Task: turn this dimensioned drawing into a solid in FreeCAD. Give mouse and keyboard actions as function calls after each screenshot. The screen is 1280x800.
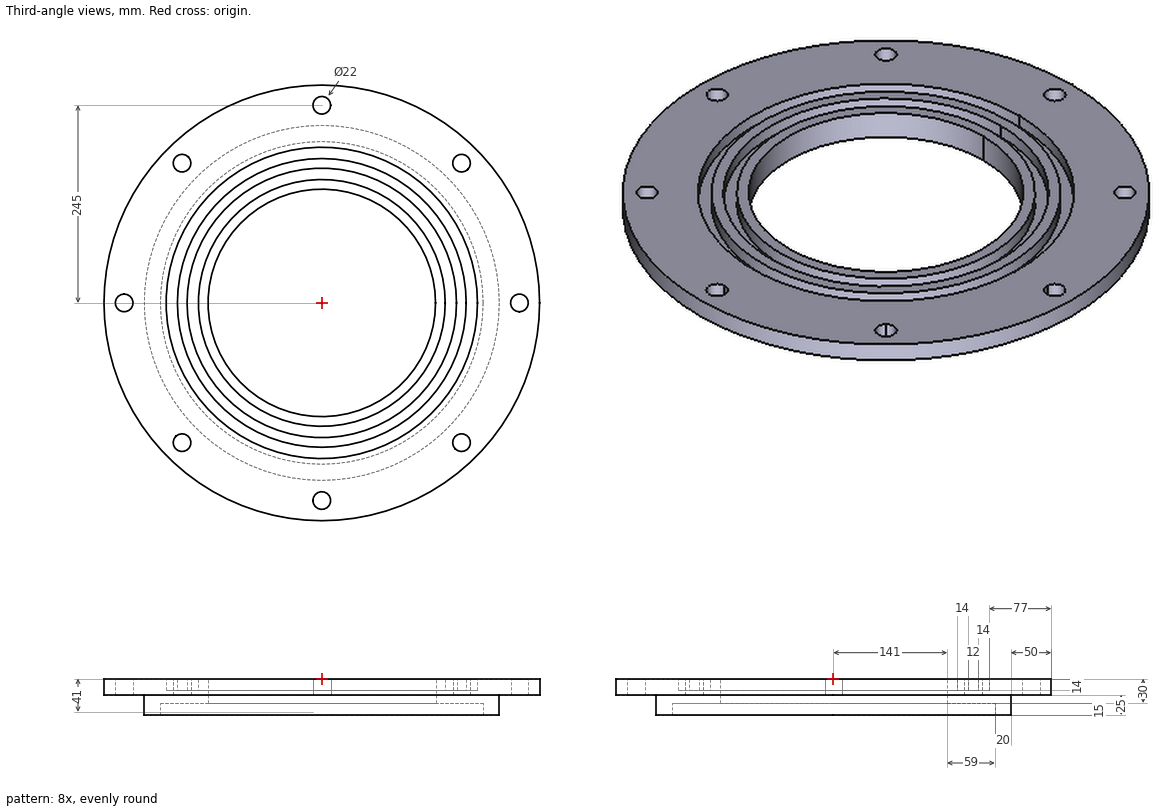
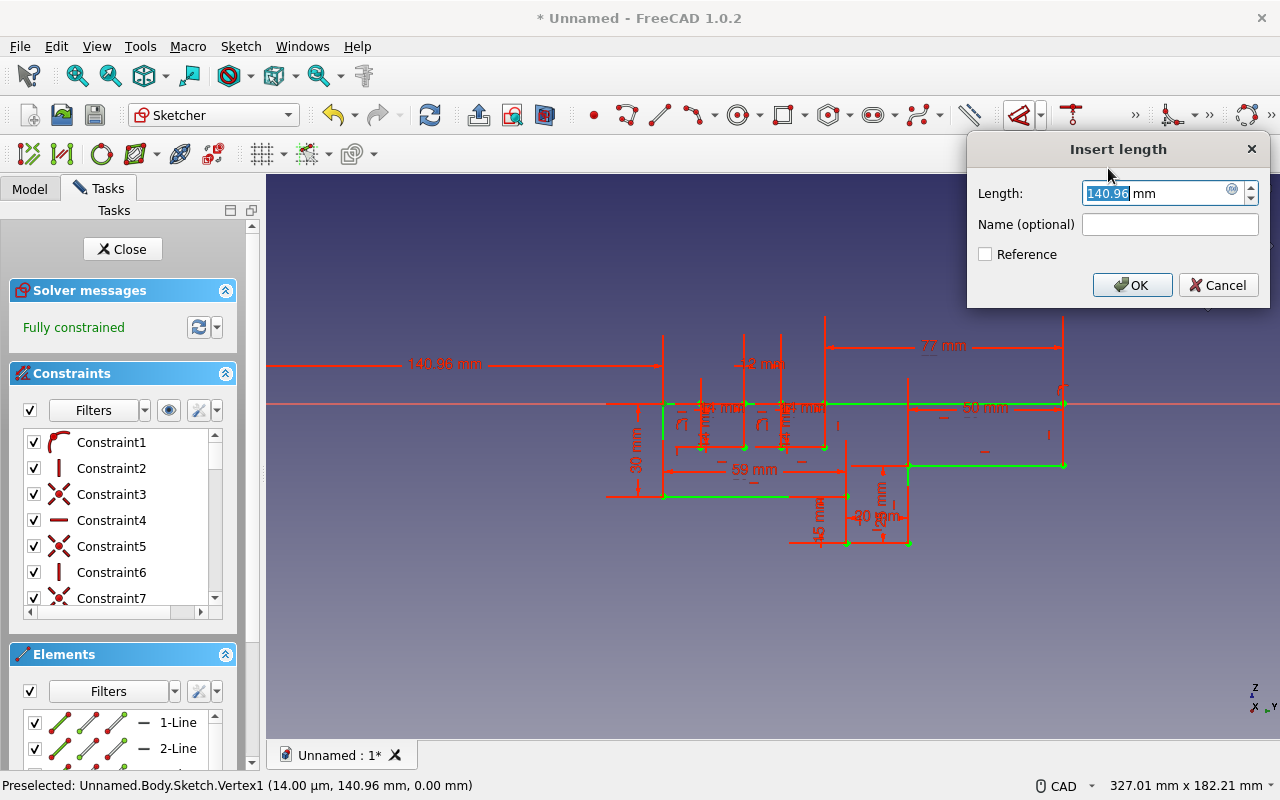
text(141)
key(Return)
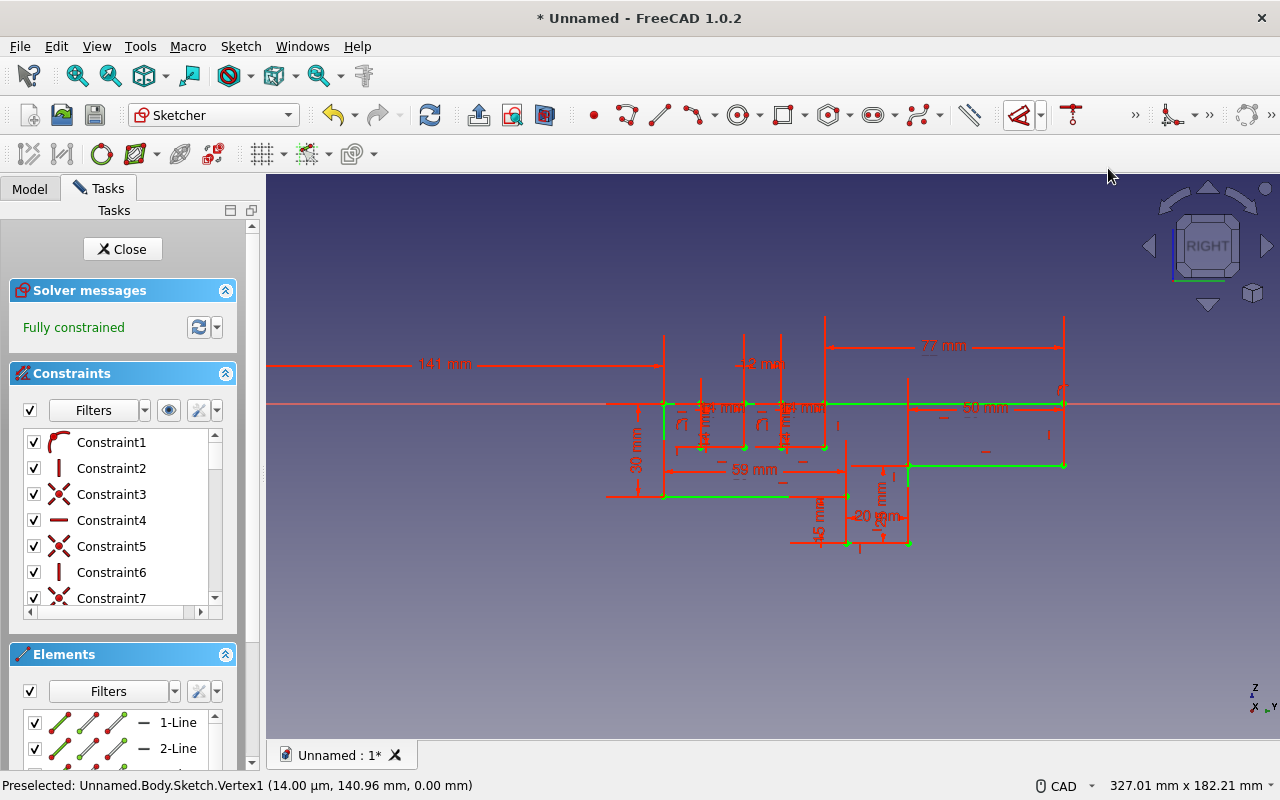
click(123, 249)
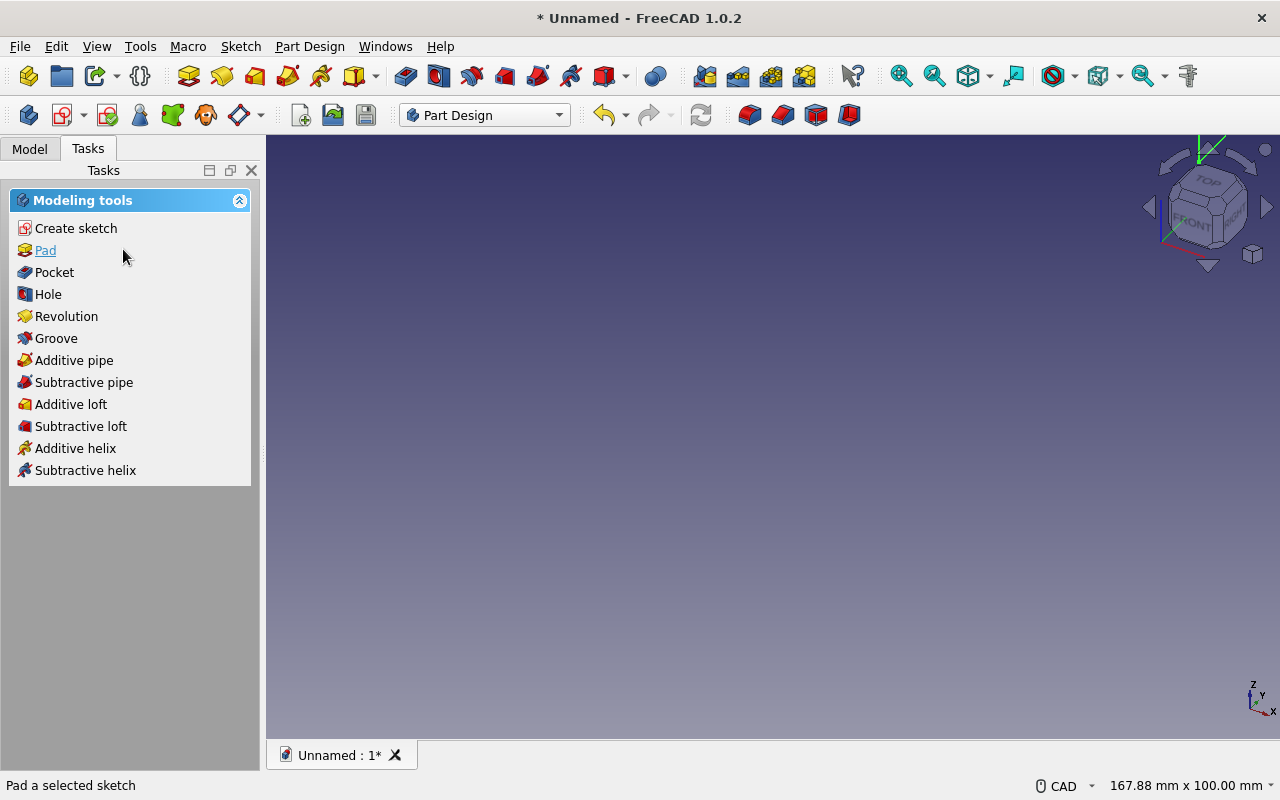
click(222, 76)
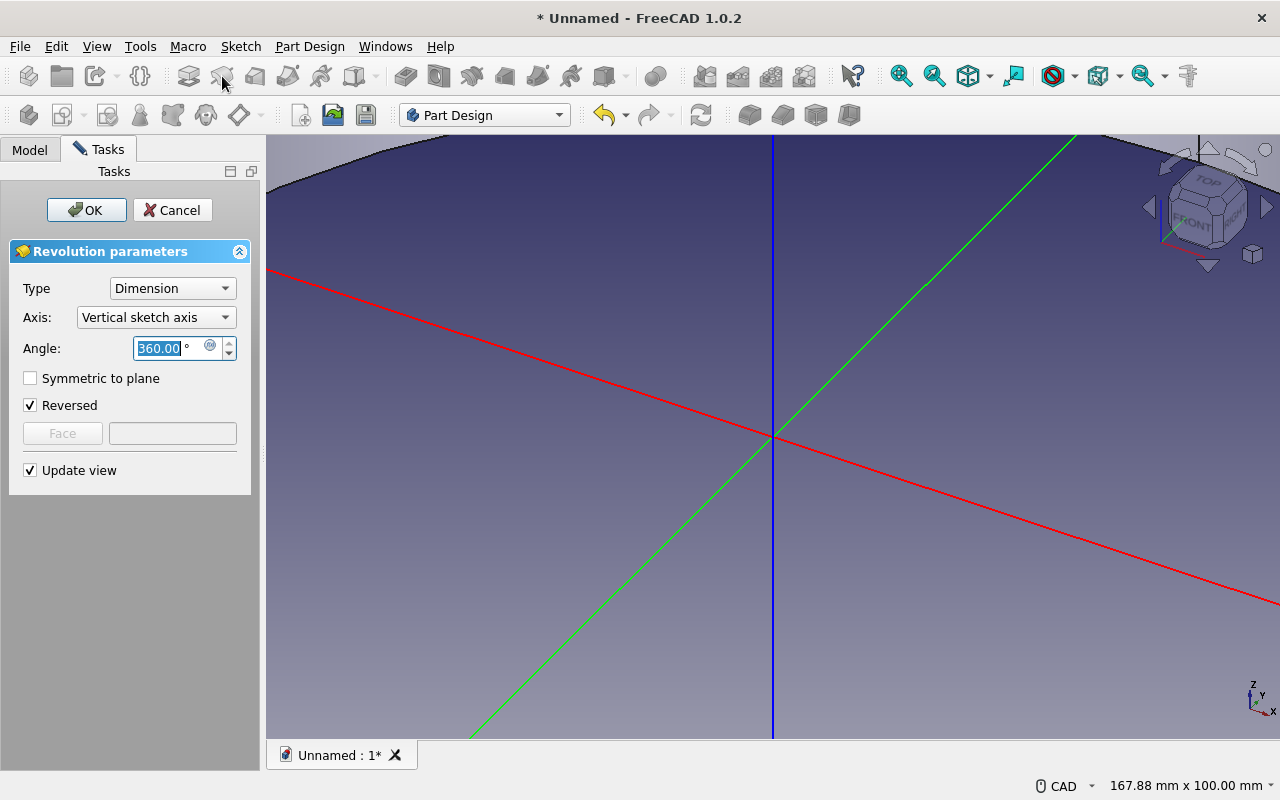
click(87, 210)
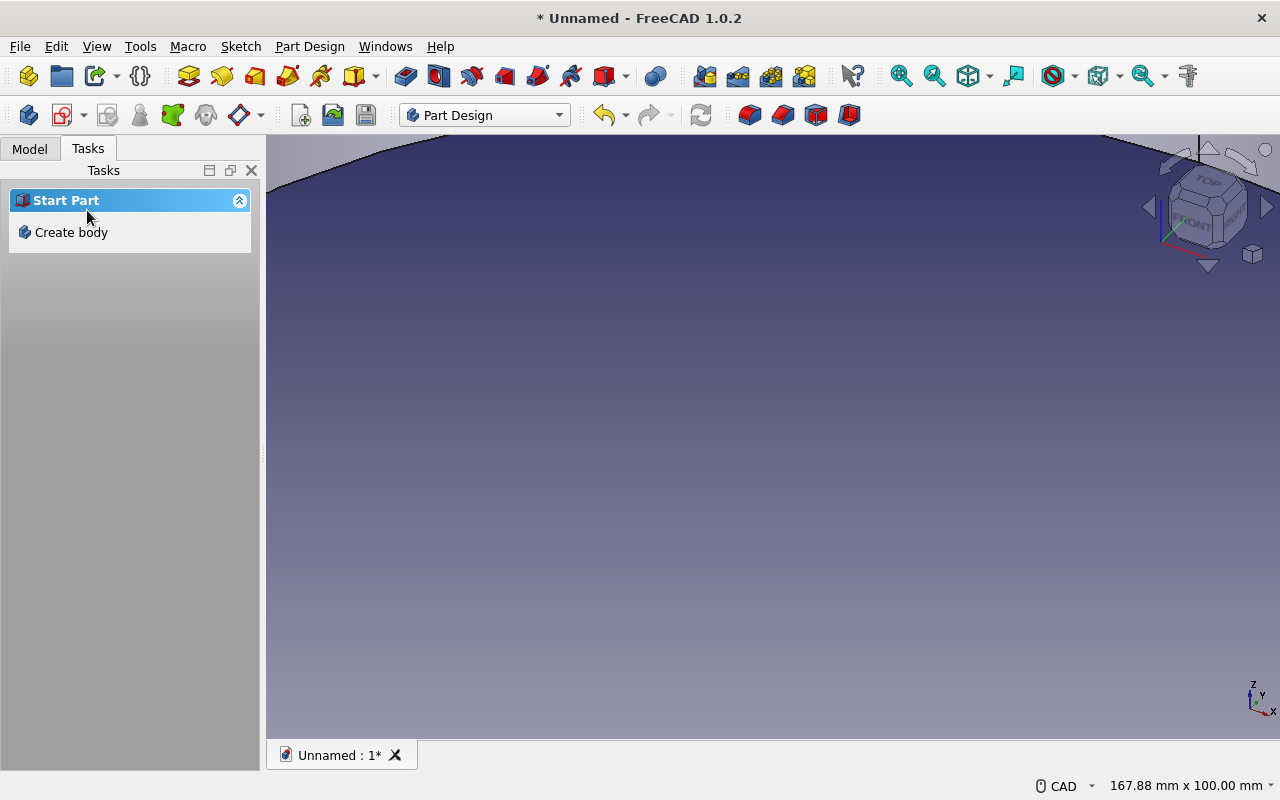
click(902, 76)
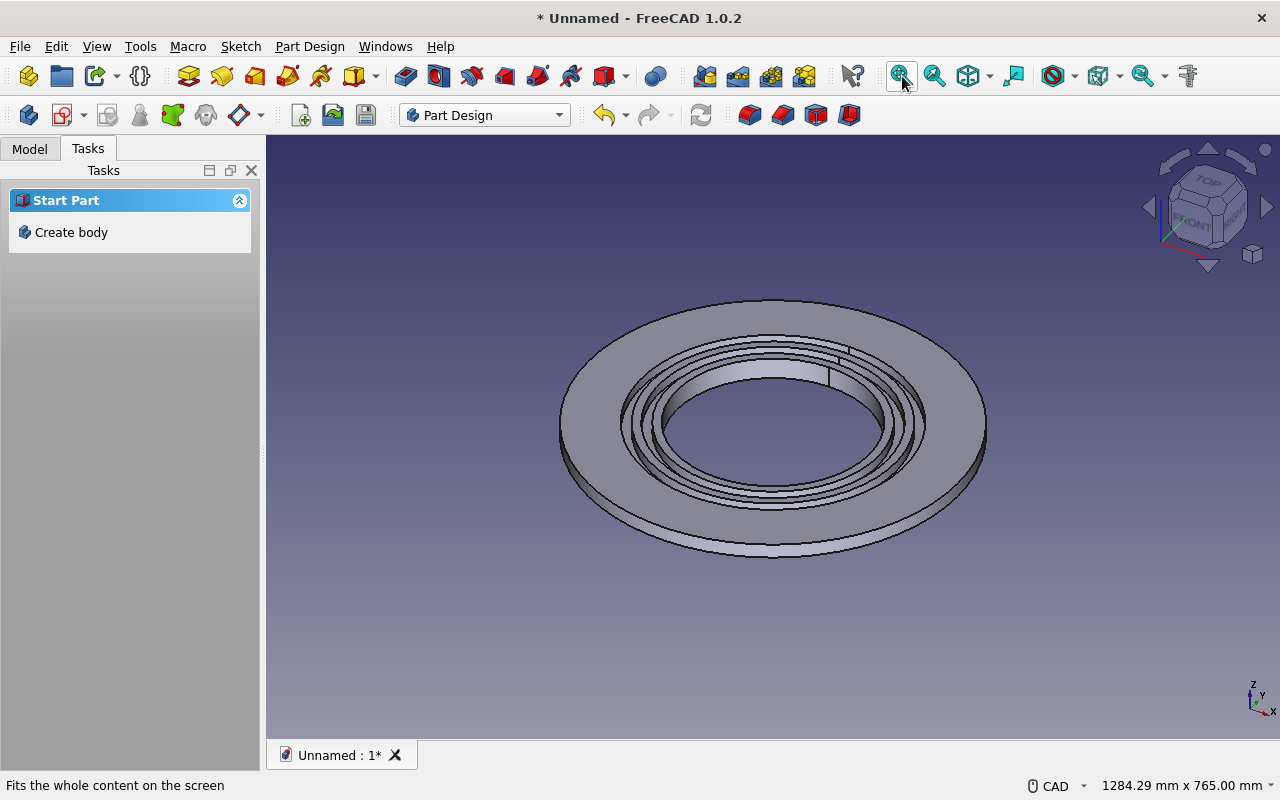
click(931, 474)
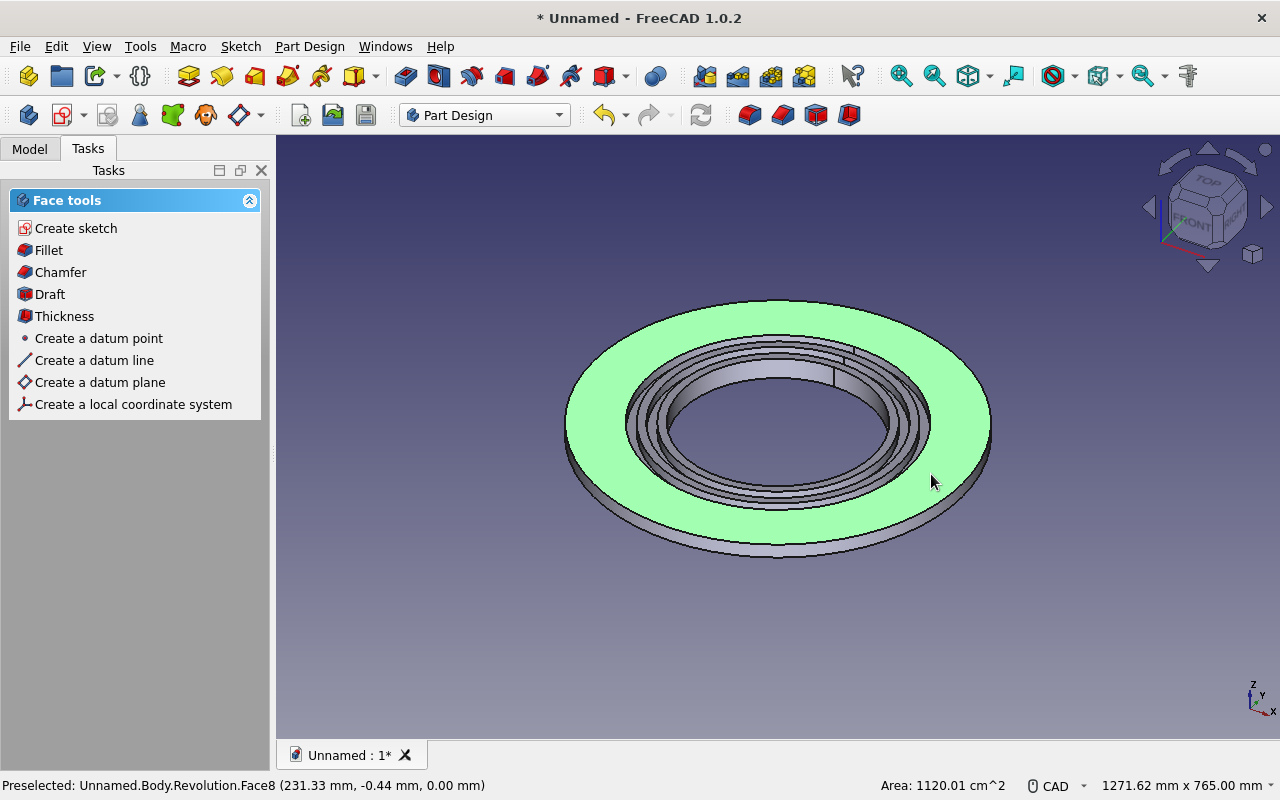
click(62, 116)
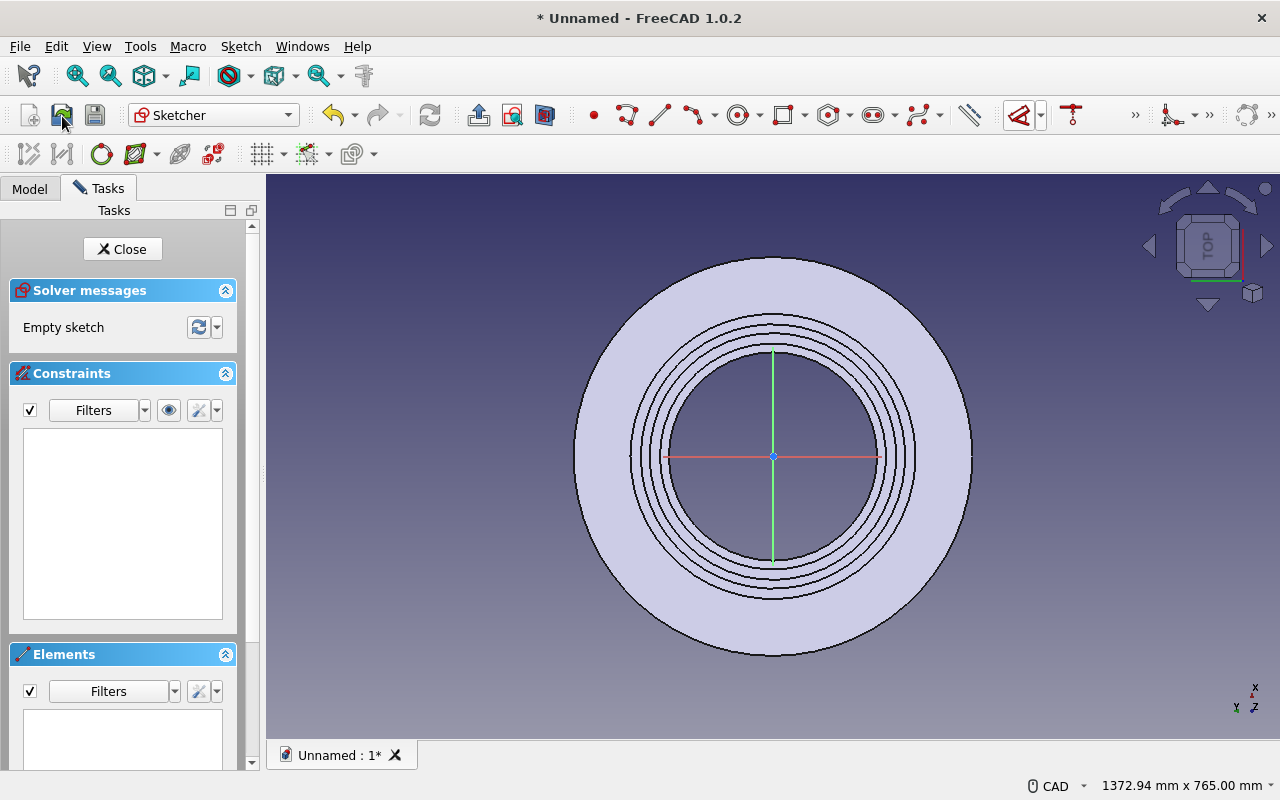
scroll(586, 457, up, 15)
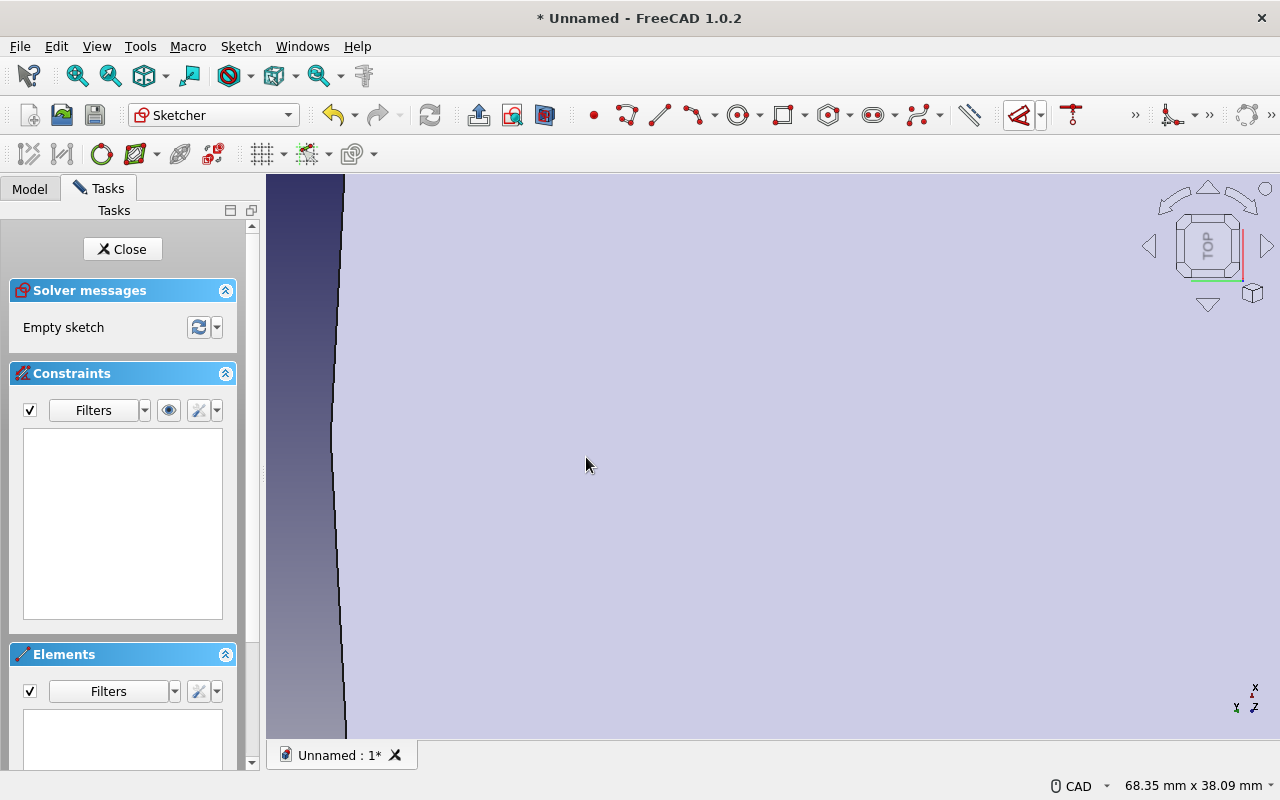
click(738, 116)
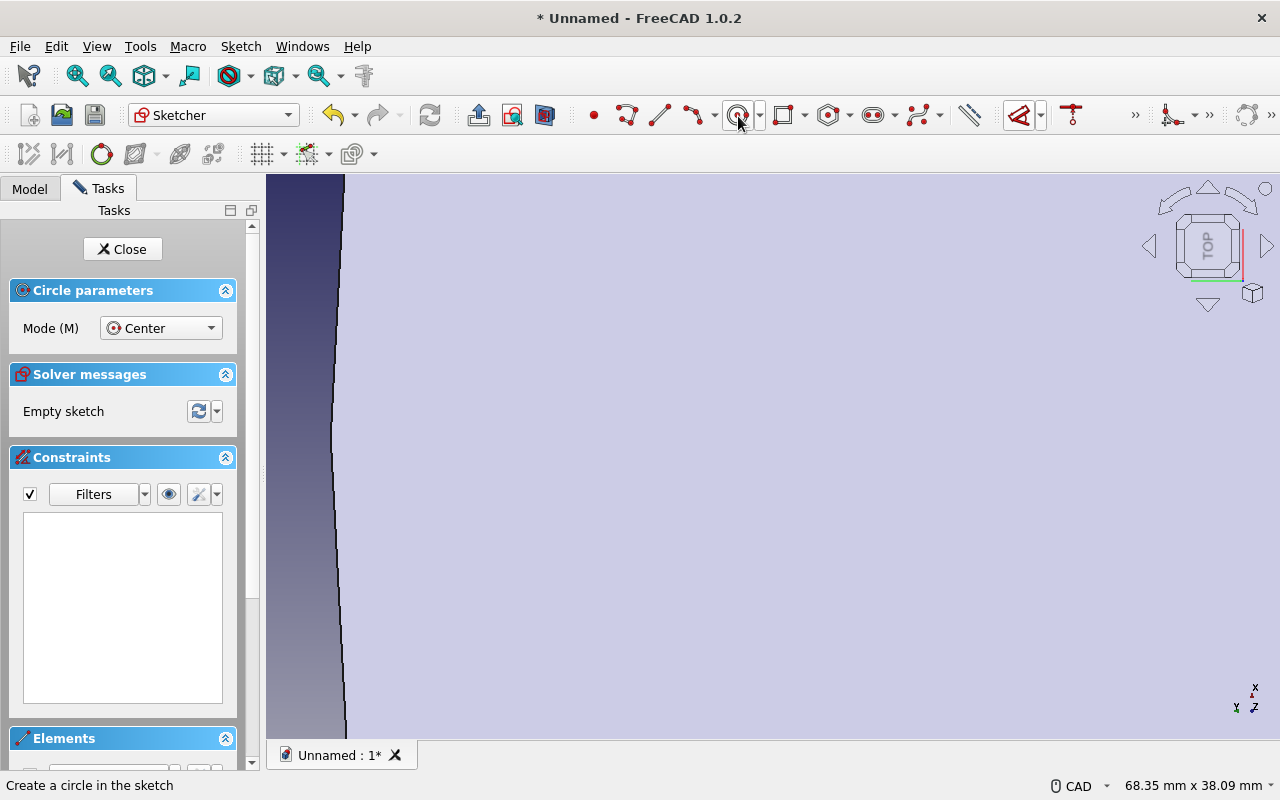
click(702, 437)
click(817, 322)
key(Escape)